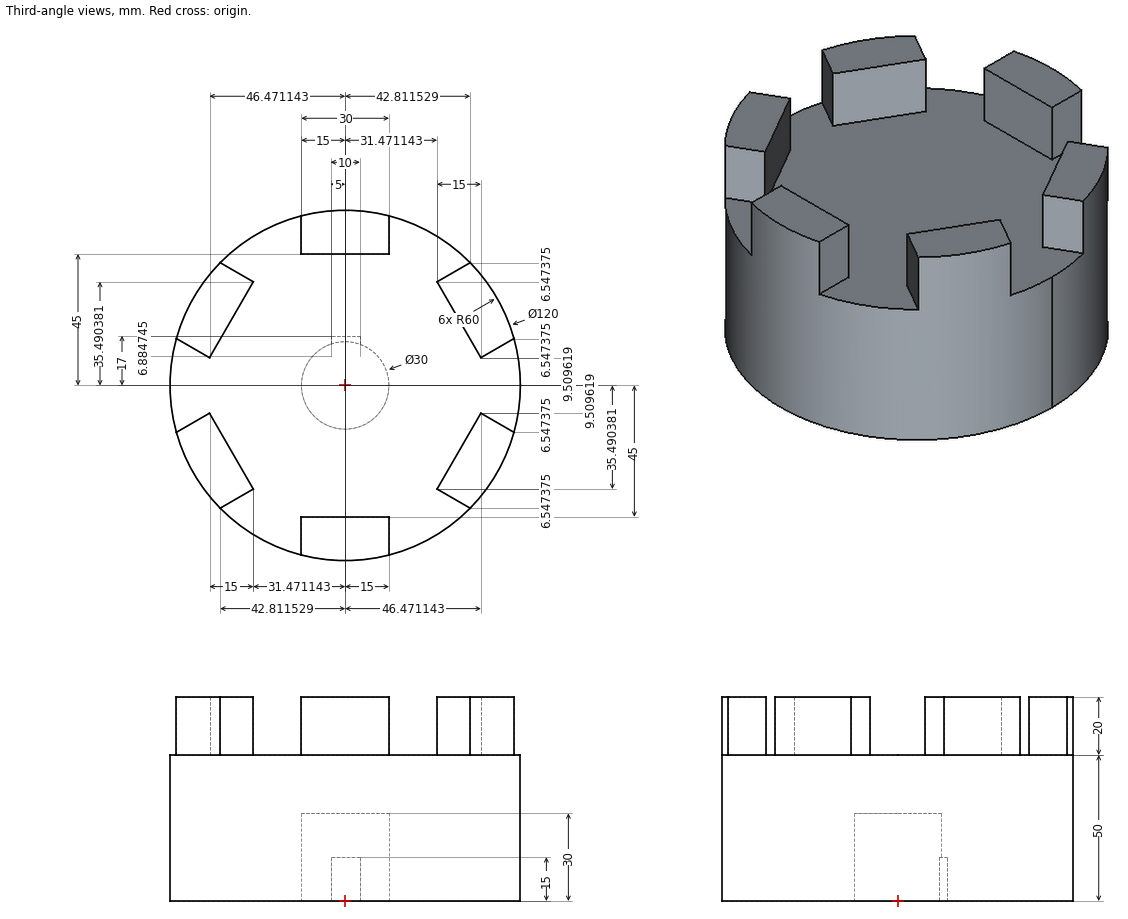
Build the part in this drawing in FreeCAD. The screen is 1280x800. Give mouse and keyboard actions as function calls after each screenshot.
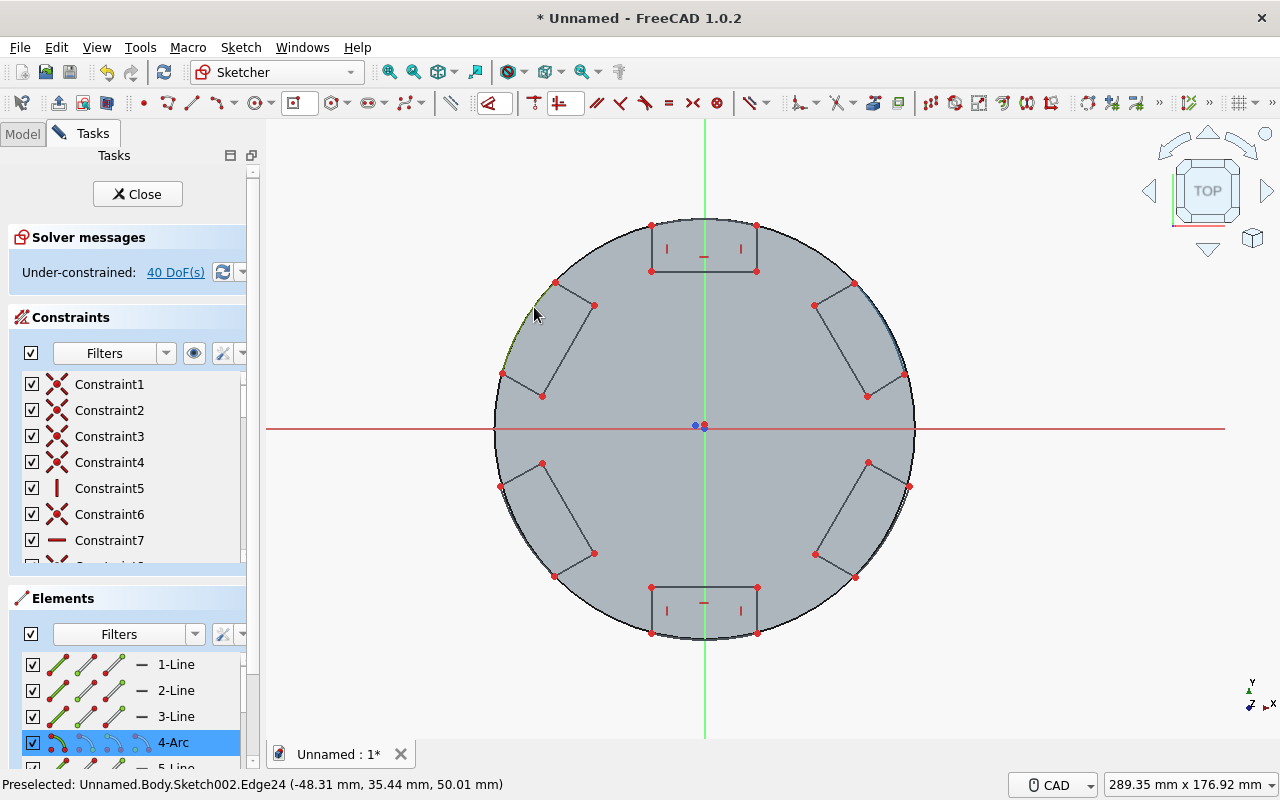
click(534, 104)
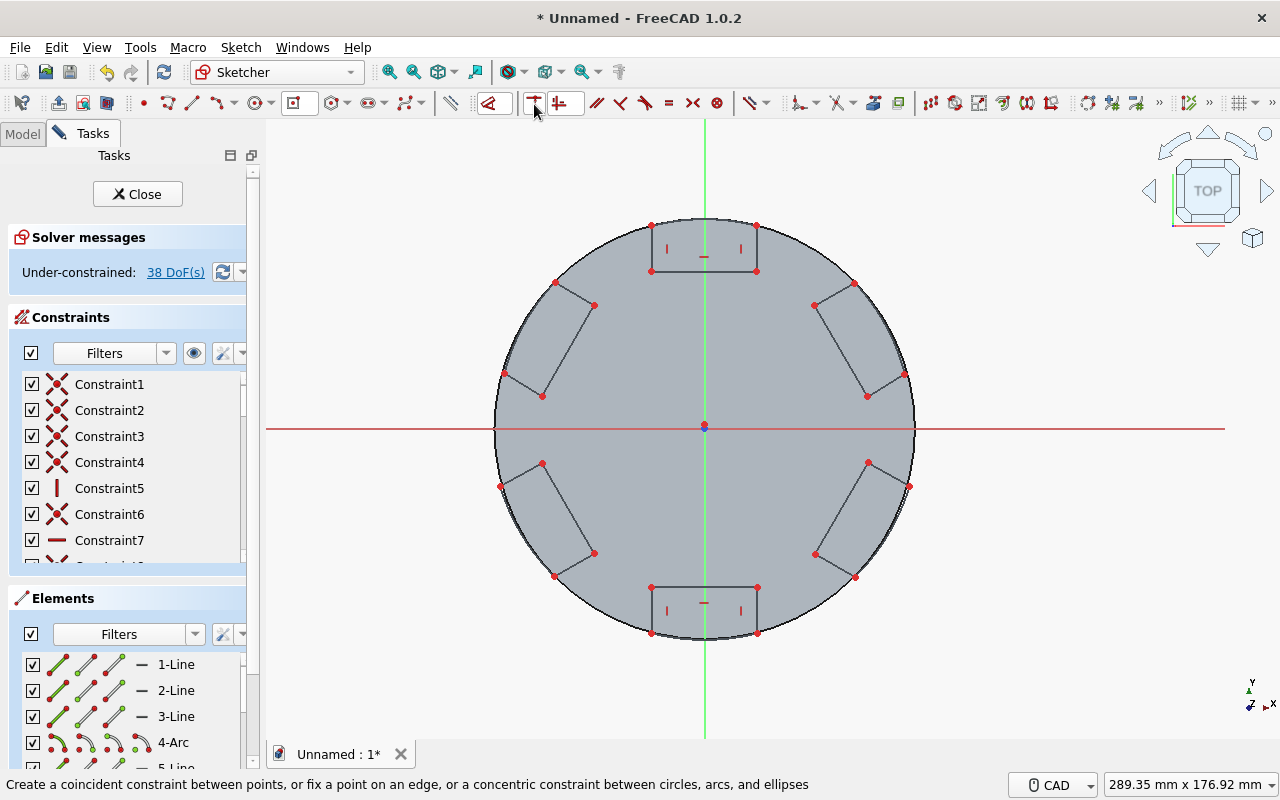
drag(695, 415, 715, 439)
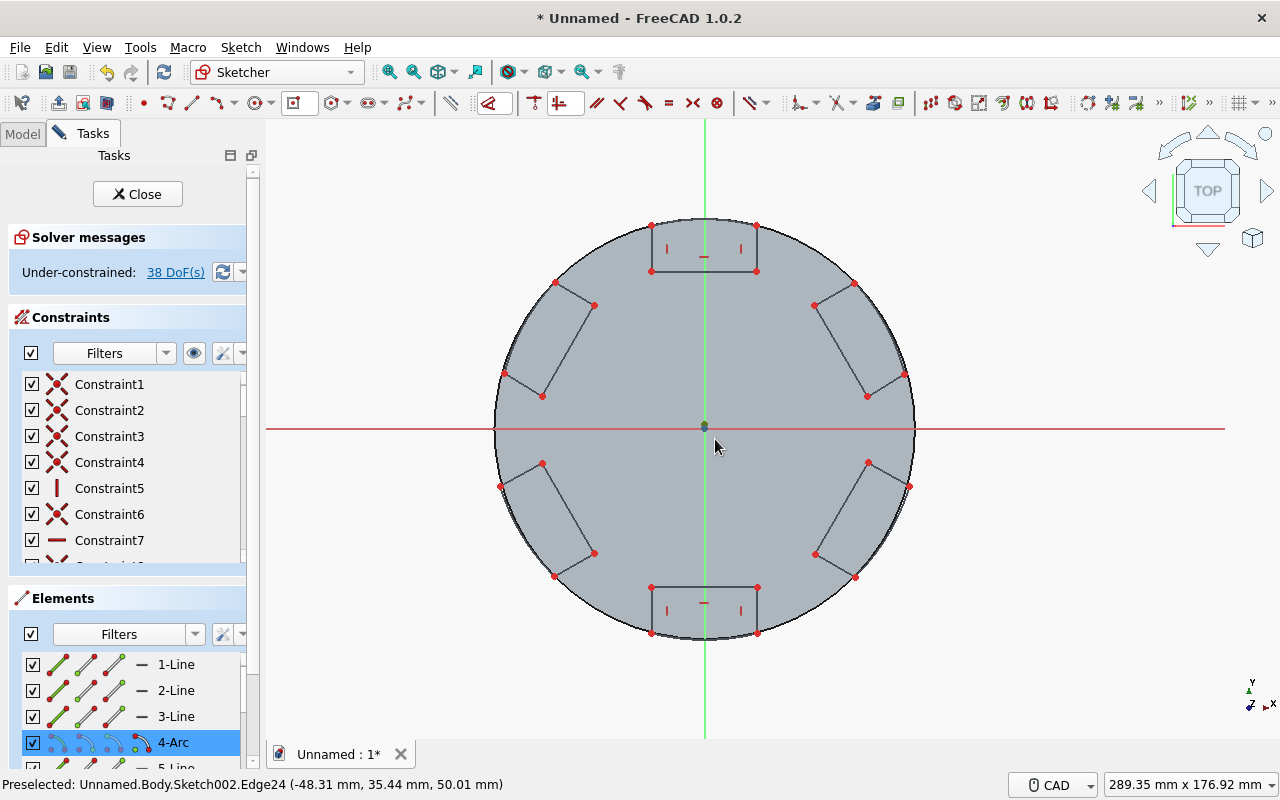
click(534, 104)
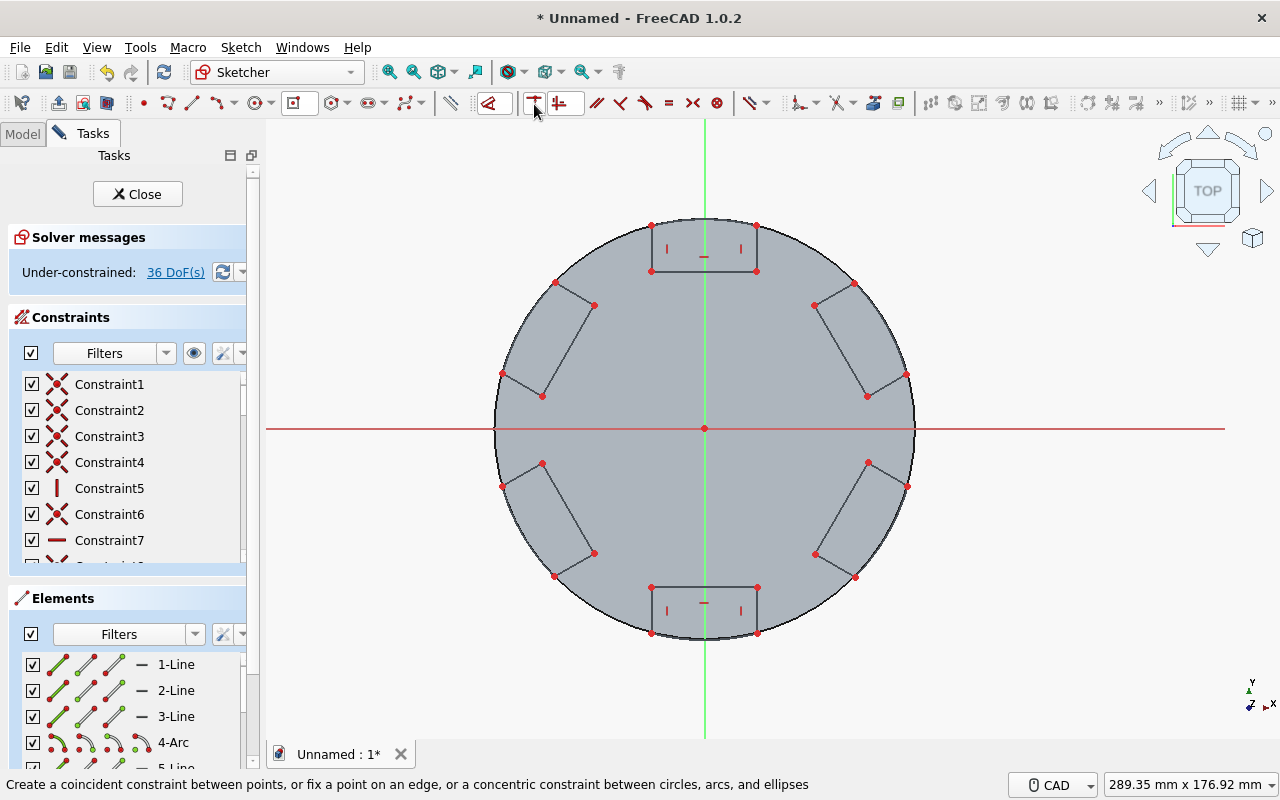
click(896, 344)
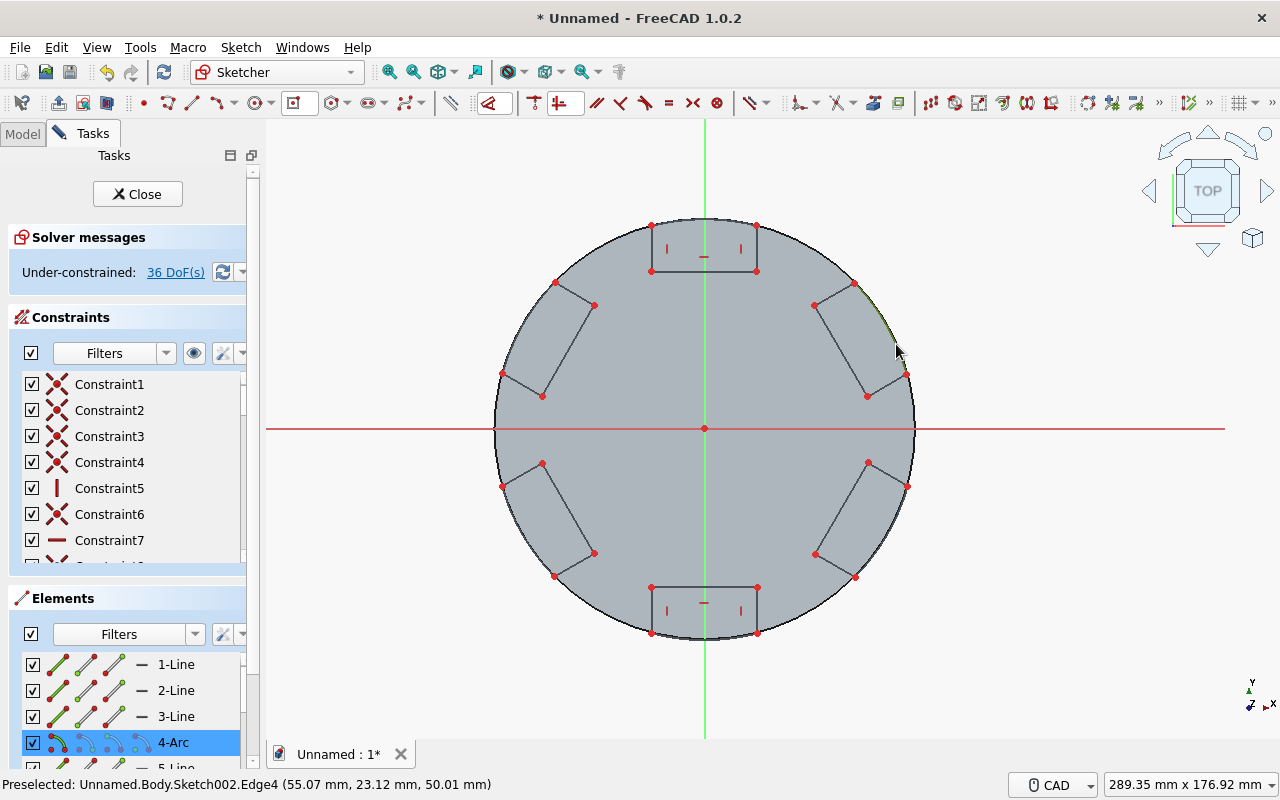
click(726, 220)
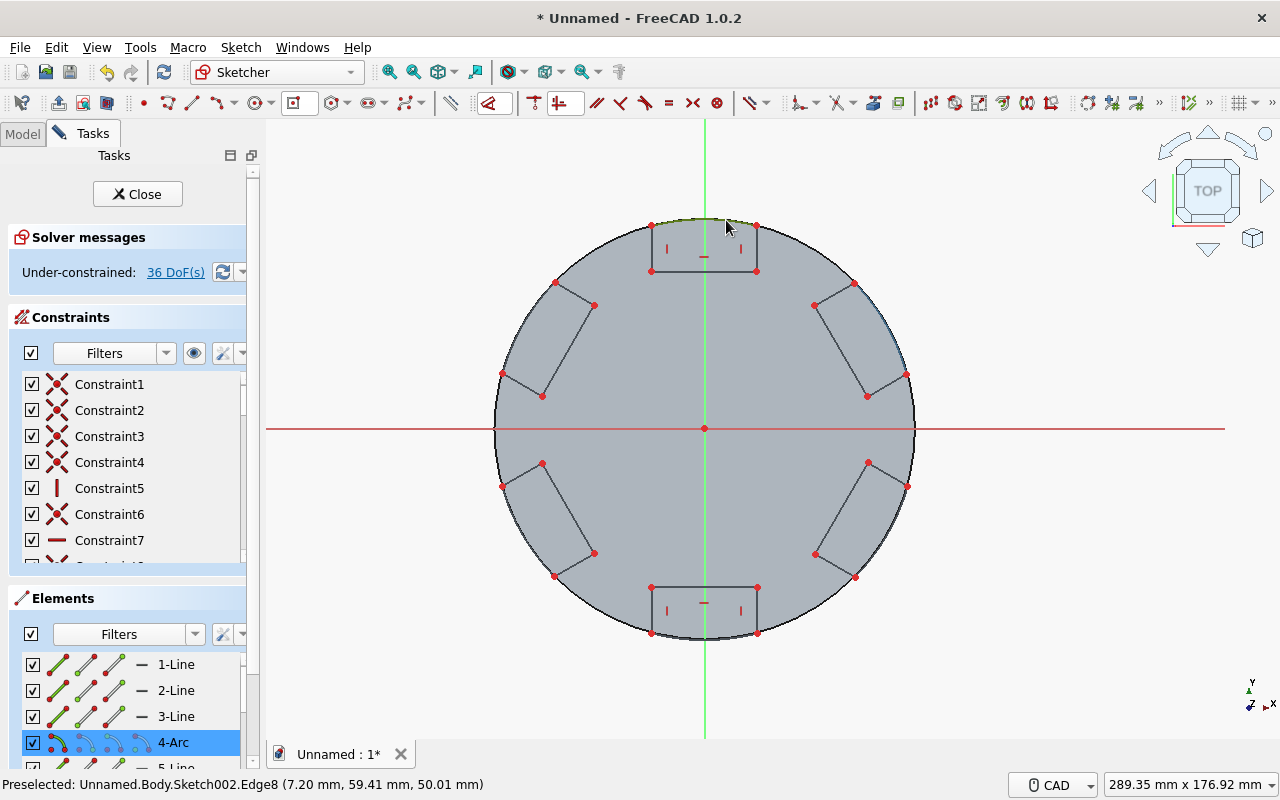
click(876, 553)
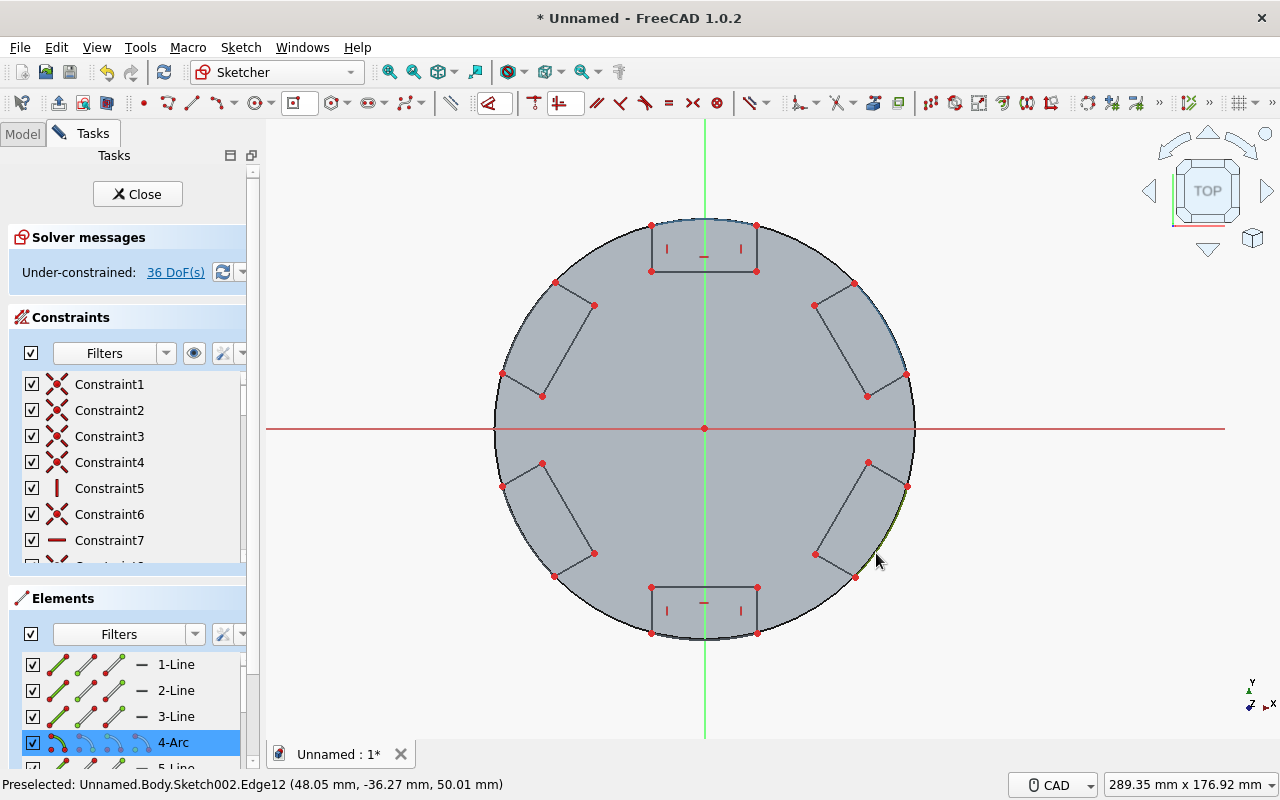
click(683, 639)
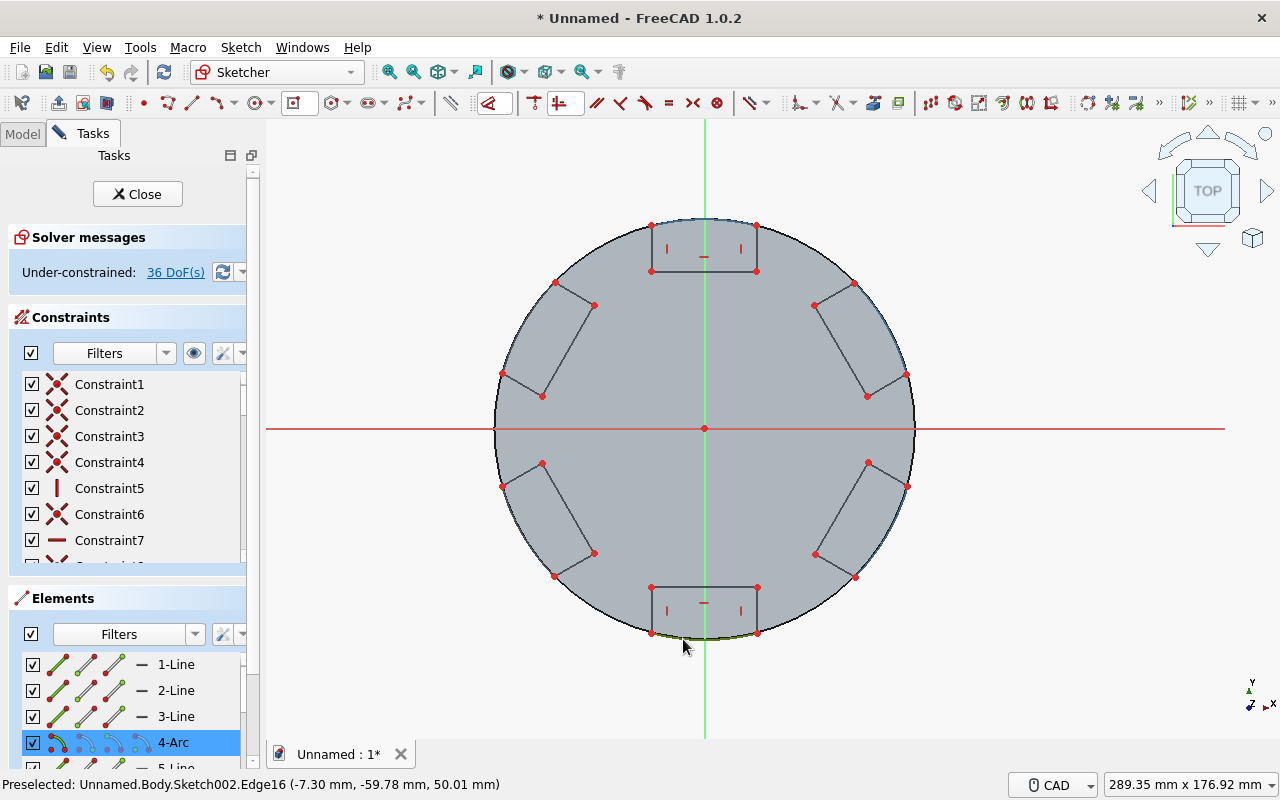
click(513, 516)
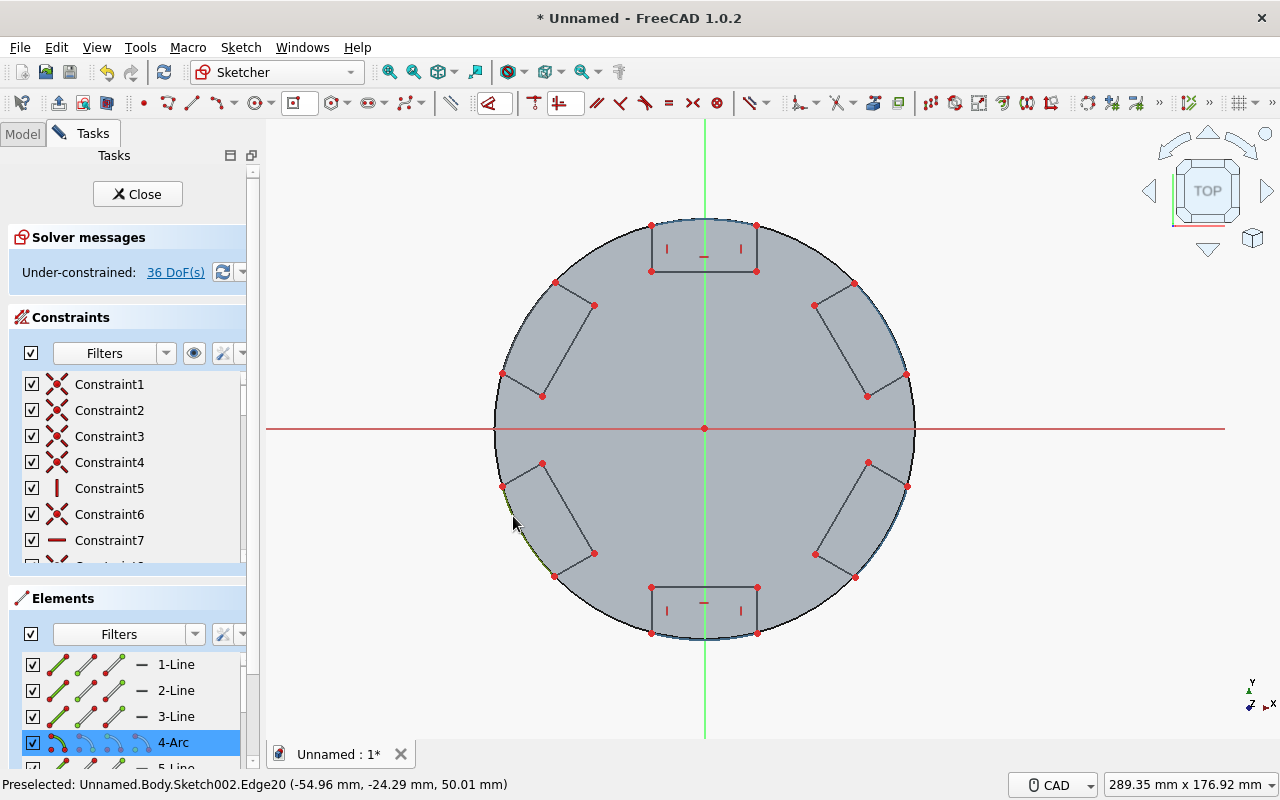
click(535, 307)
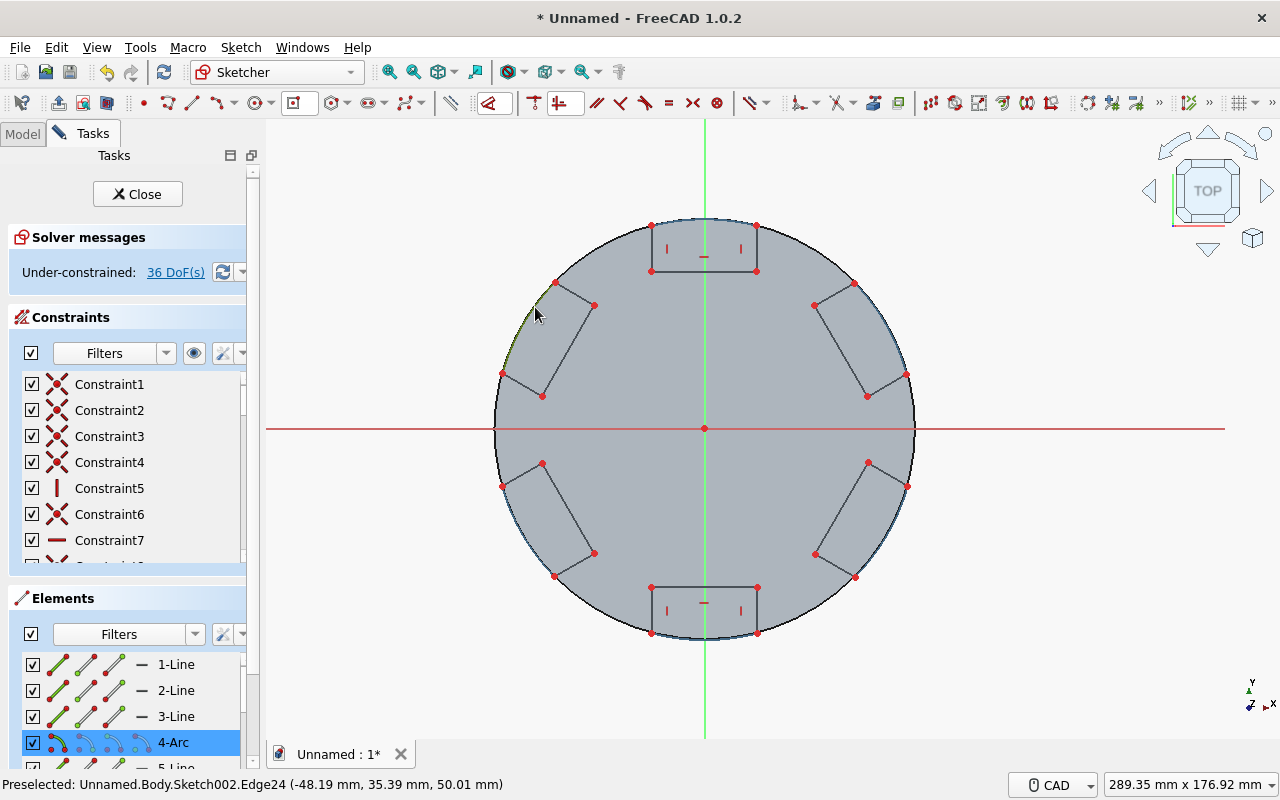
key(e)